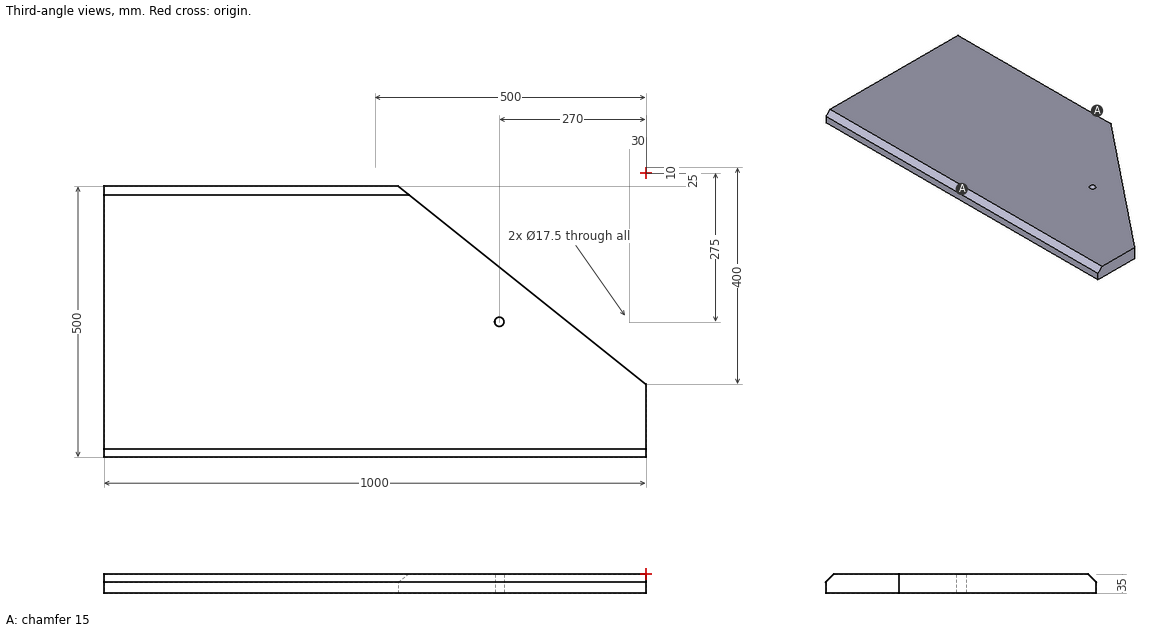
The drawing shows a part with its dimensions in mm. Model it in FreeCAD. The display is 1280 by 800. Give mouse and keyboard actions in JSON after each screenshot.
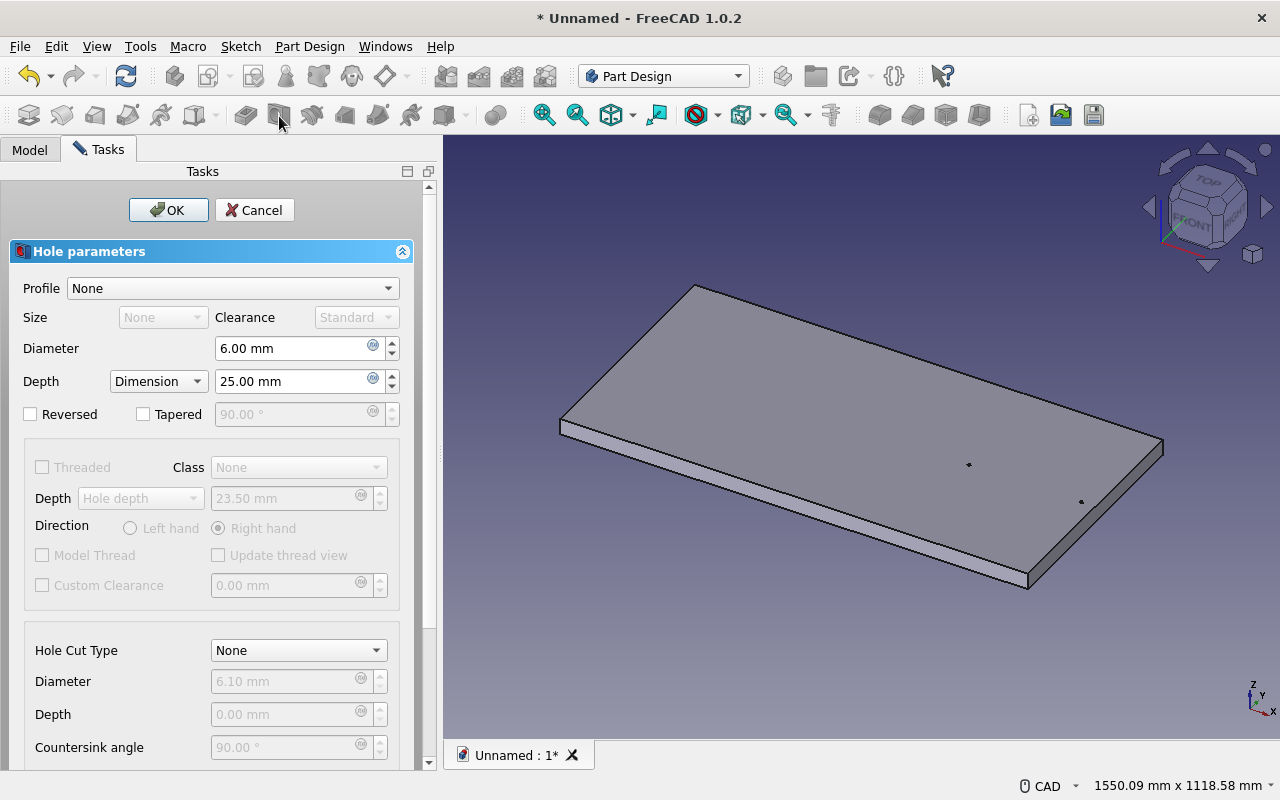
{"action": "triple_click", "coordinate": [300, 348]}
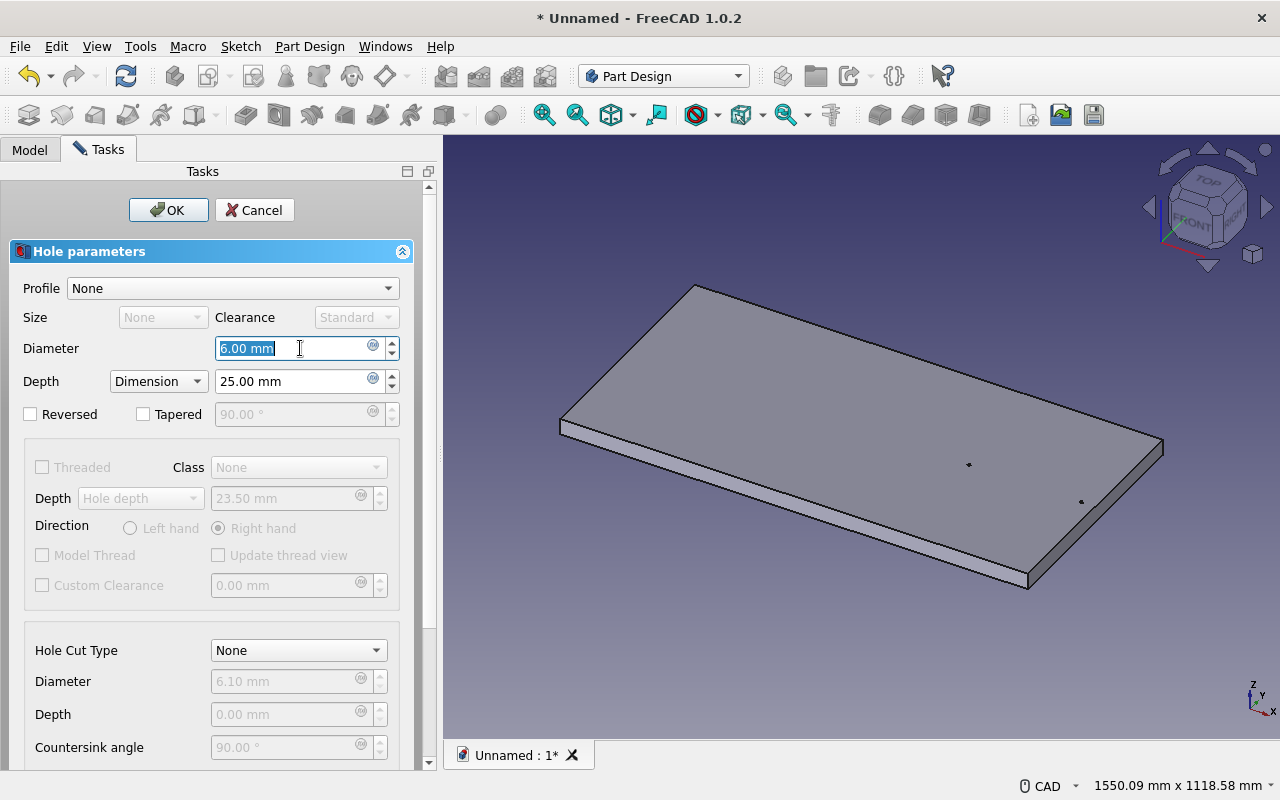
{"action": "type", "text": "17.5"}
{"action": "key", "text": "Tab"}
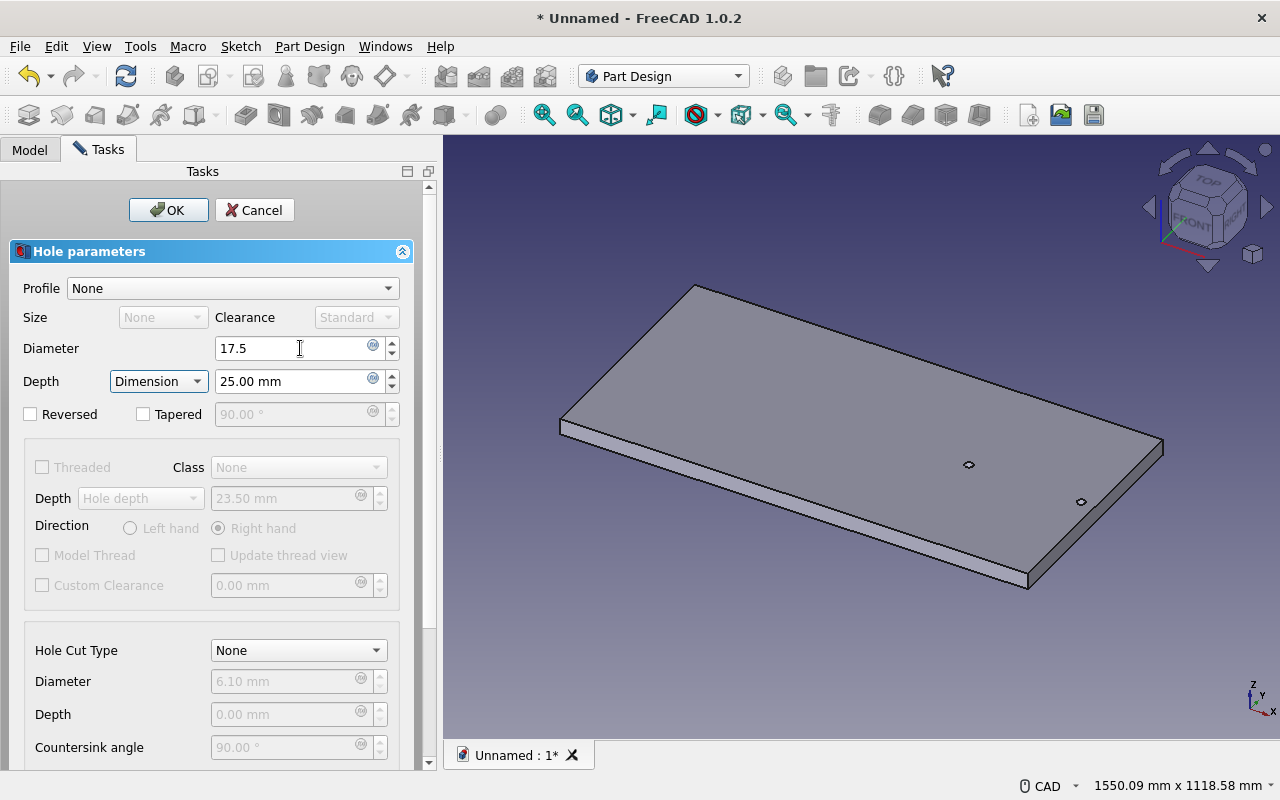
{"action": "left_click", "coordinate": [160, 382]}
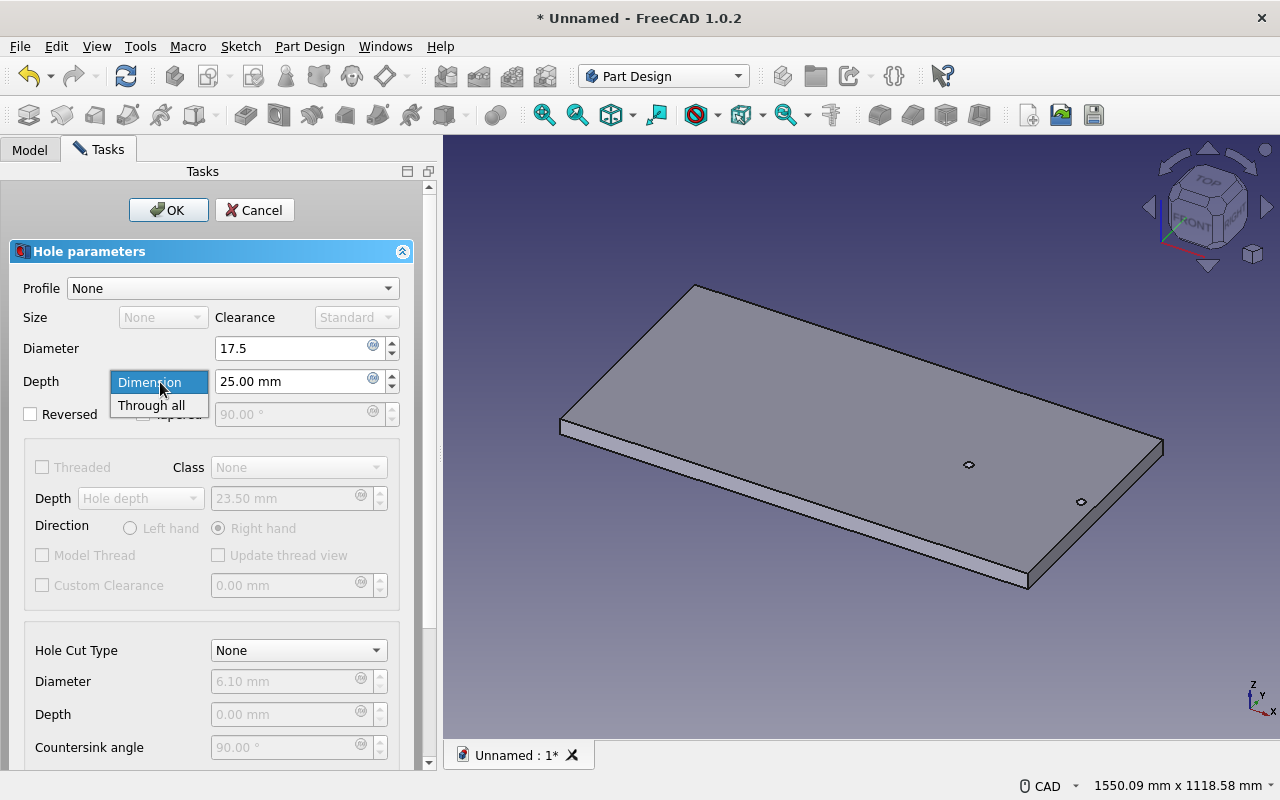
{"action": "left_click", "coordinate": [158, 406]}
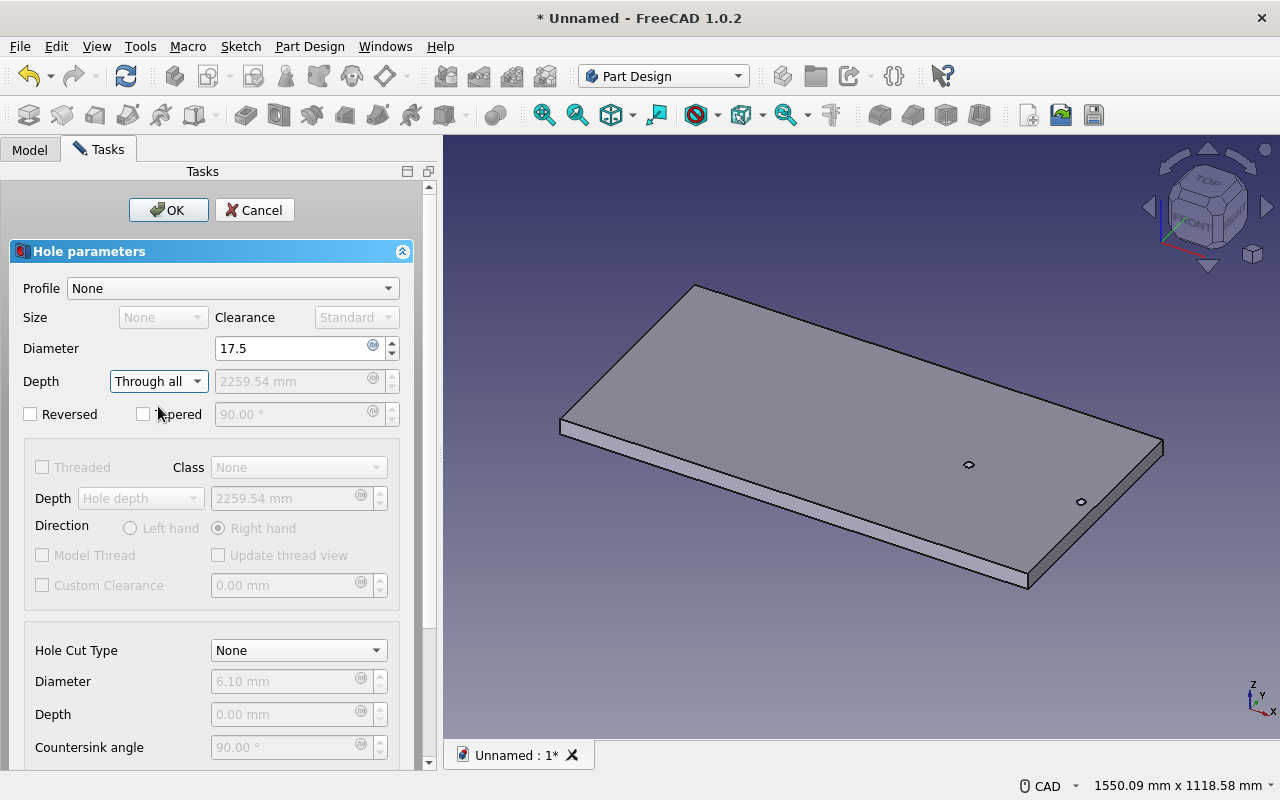
{"action": "left_click", "coordinate": [169, 210]}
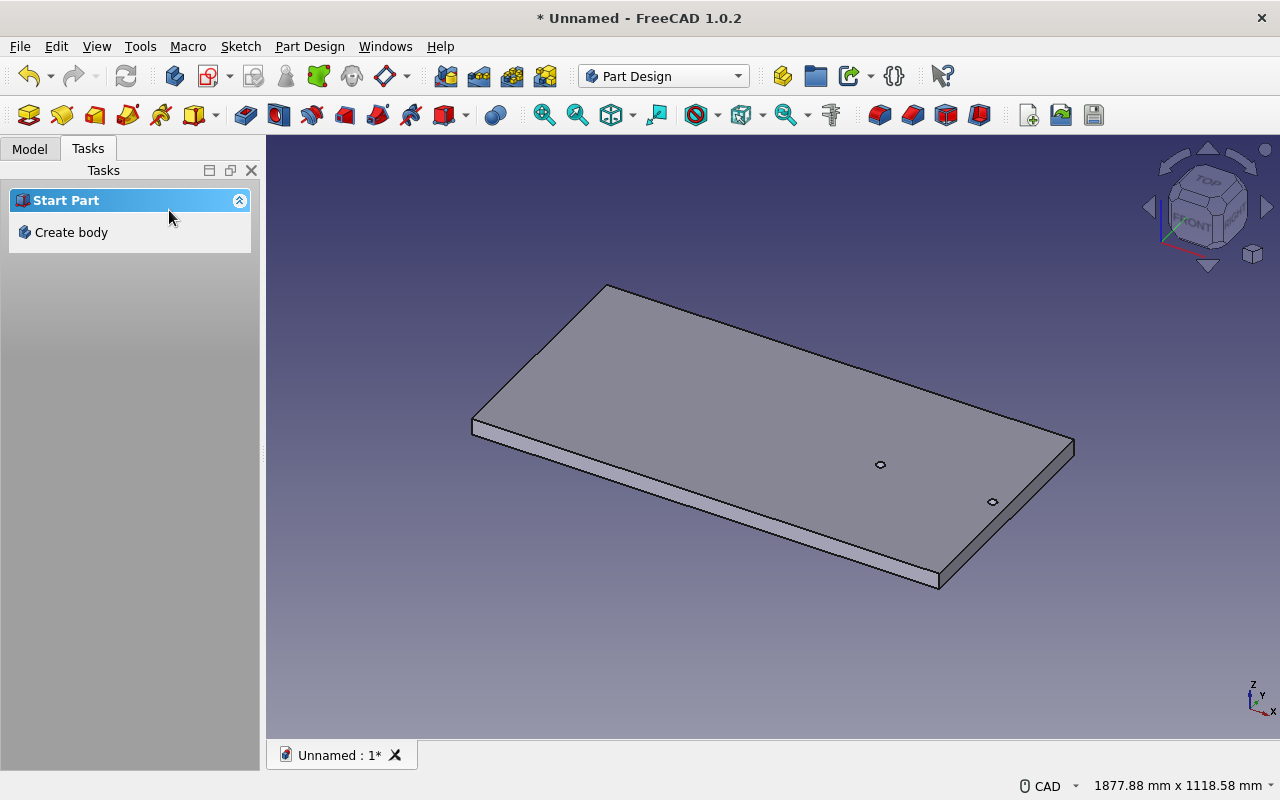
{"action": "left_click", "coordinate": [706, 495]}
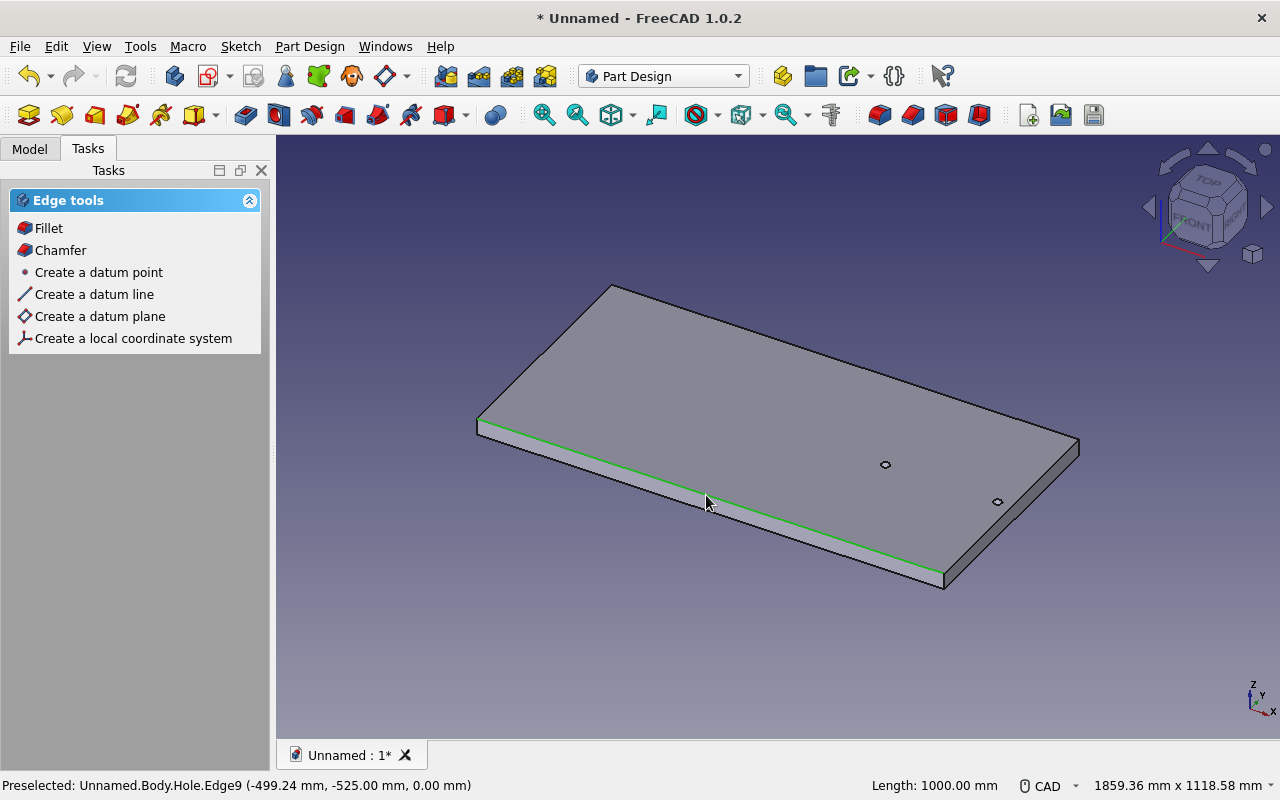
{"action": "key", "text": "0"}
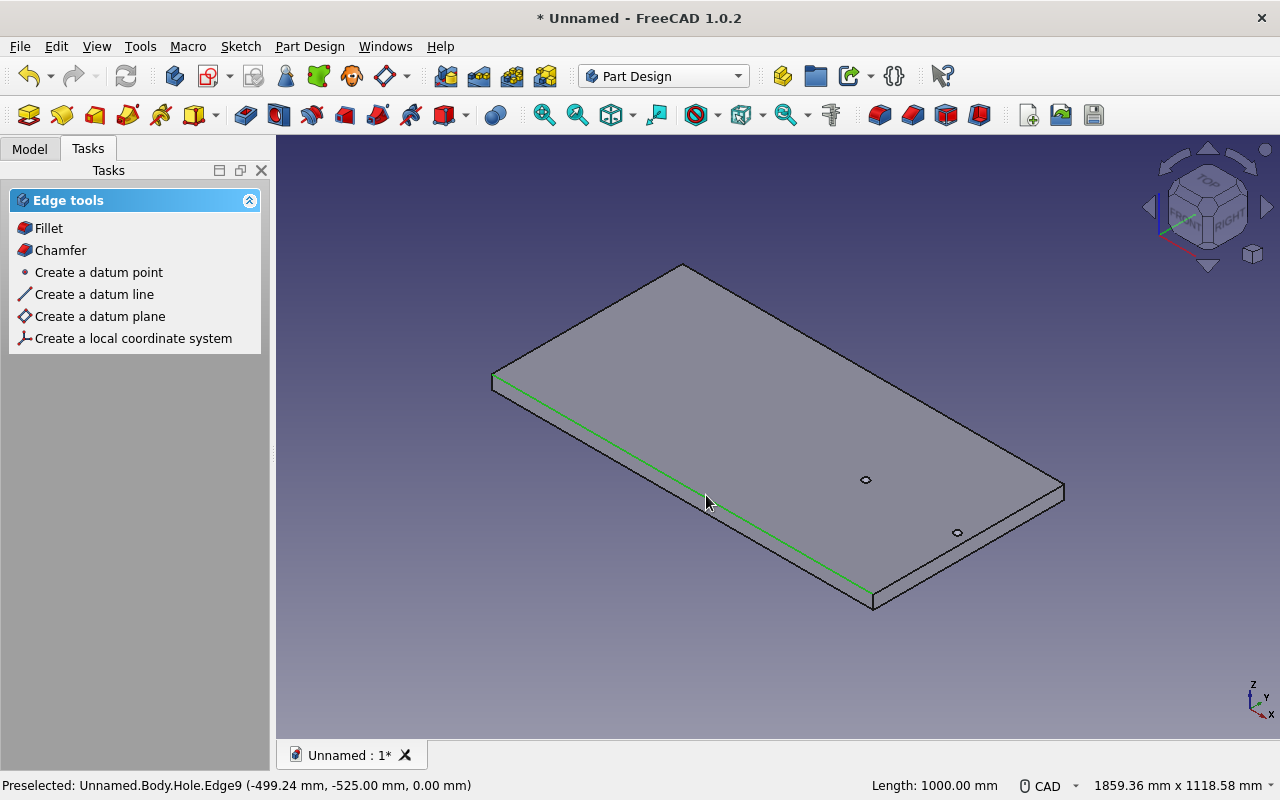
{"action": "key", "text": "2"}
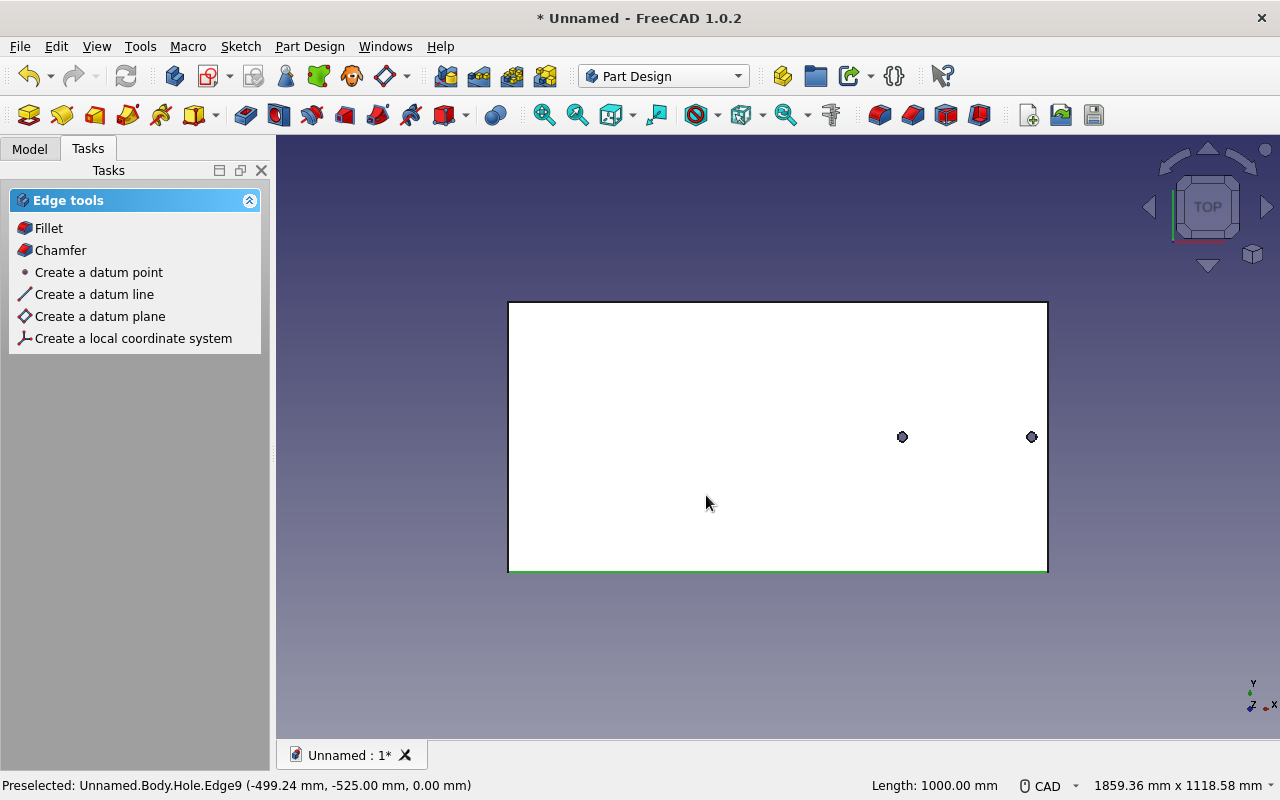
{"action": "left_click", "coordinate": [778, 301], "text": "ctrl"}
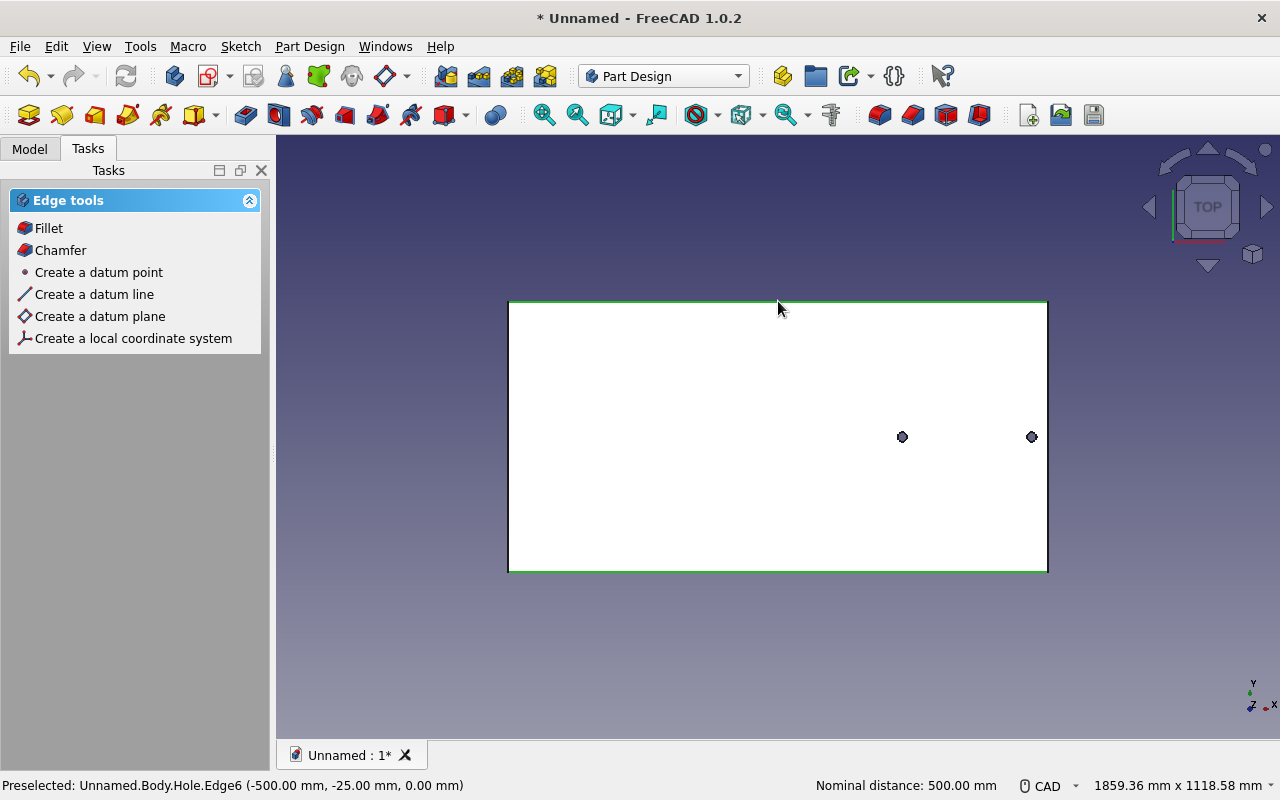
{"action": "left_click", "coordinate": [913, 116]}